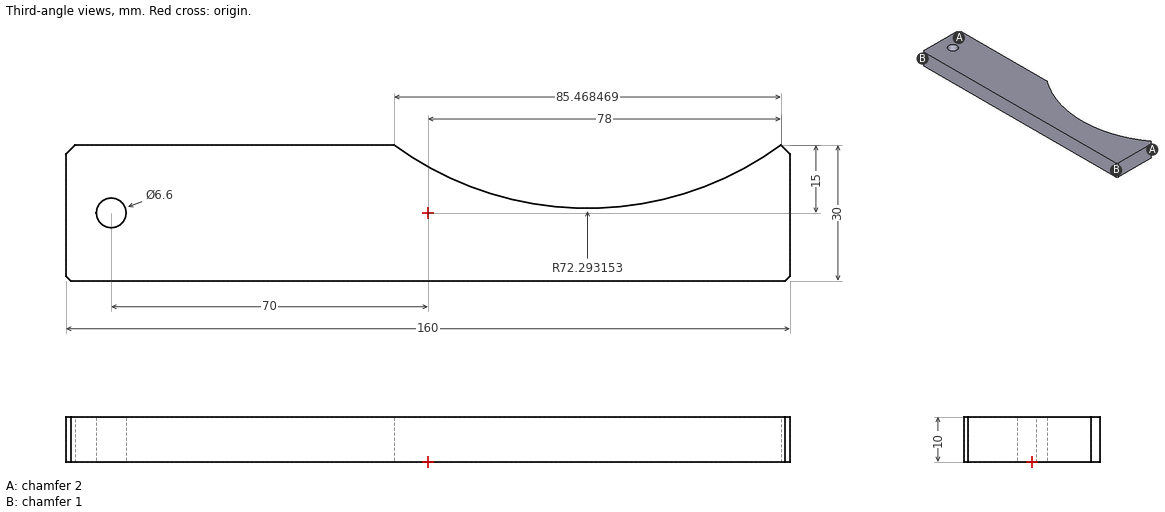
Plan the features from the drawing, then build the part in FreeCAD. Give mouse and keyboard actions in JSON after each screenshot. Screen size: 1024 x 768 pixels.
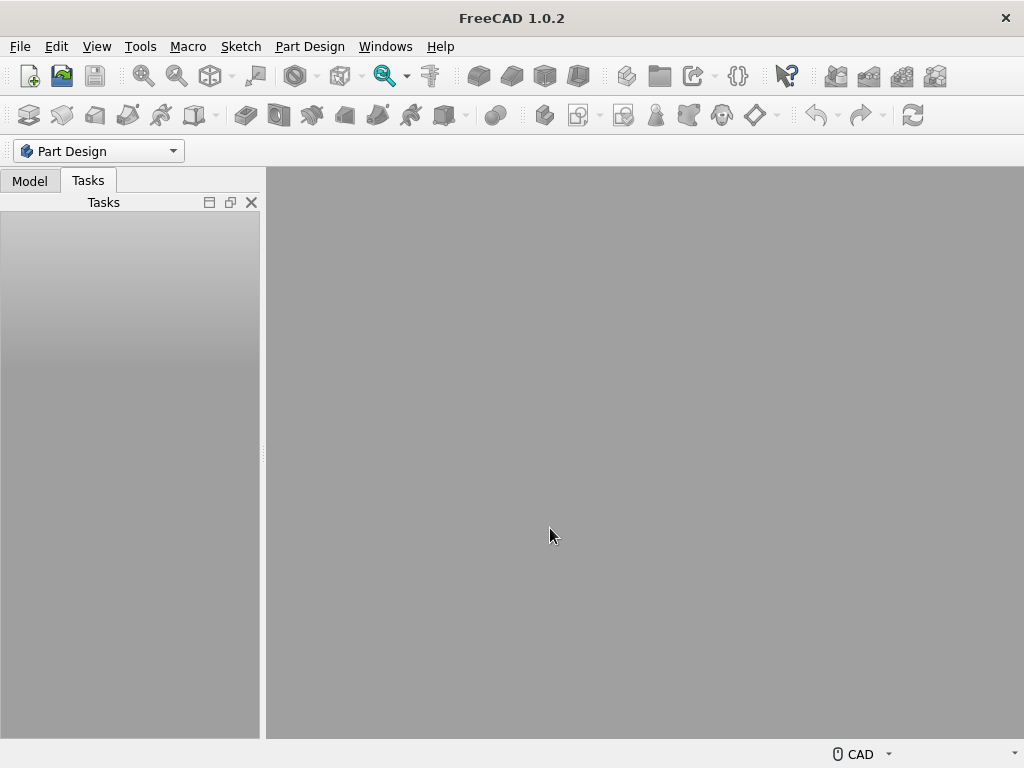
{"action": "left_click", "coordinate": [29, 76]}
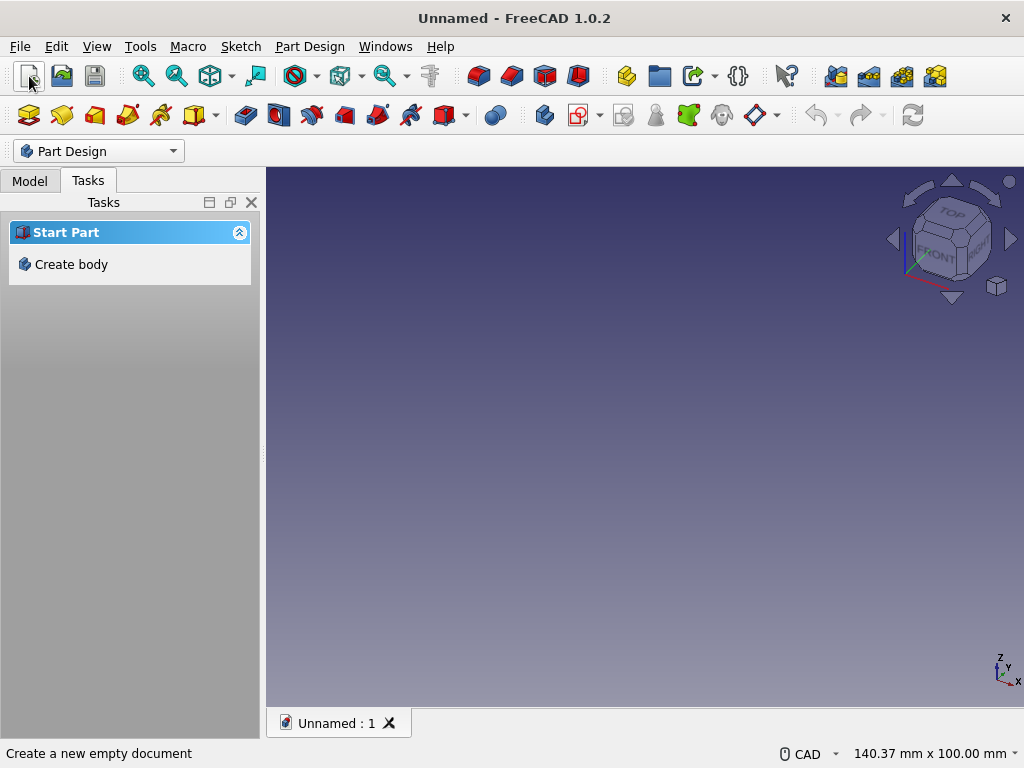
{"action": "left_click", "coordinate": [578, 116]}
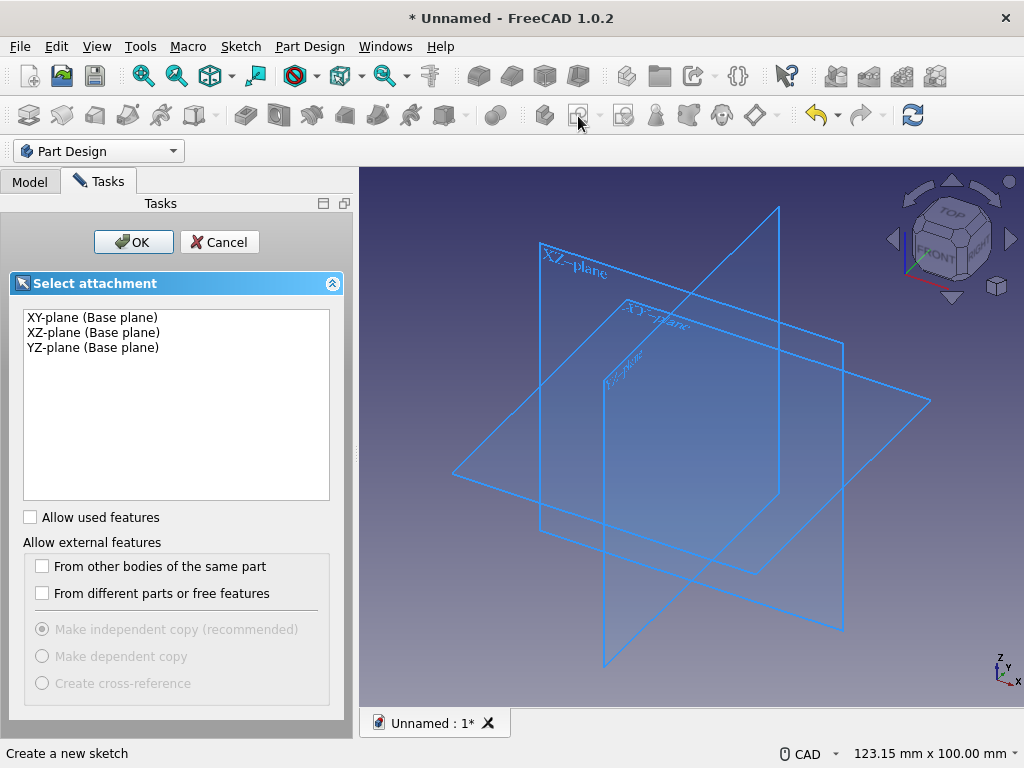
{"action": "left_click", "coordinate": [84, 318]}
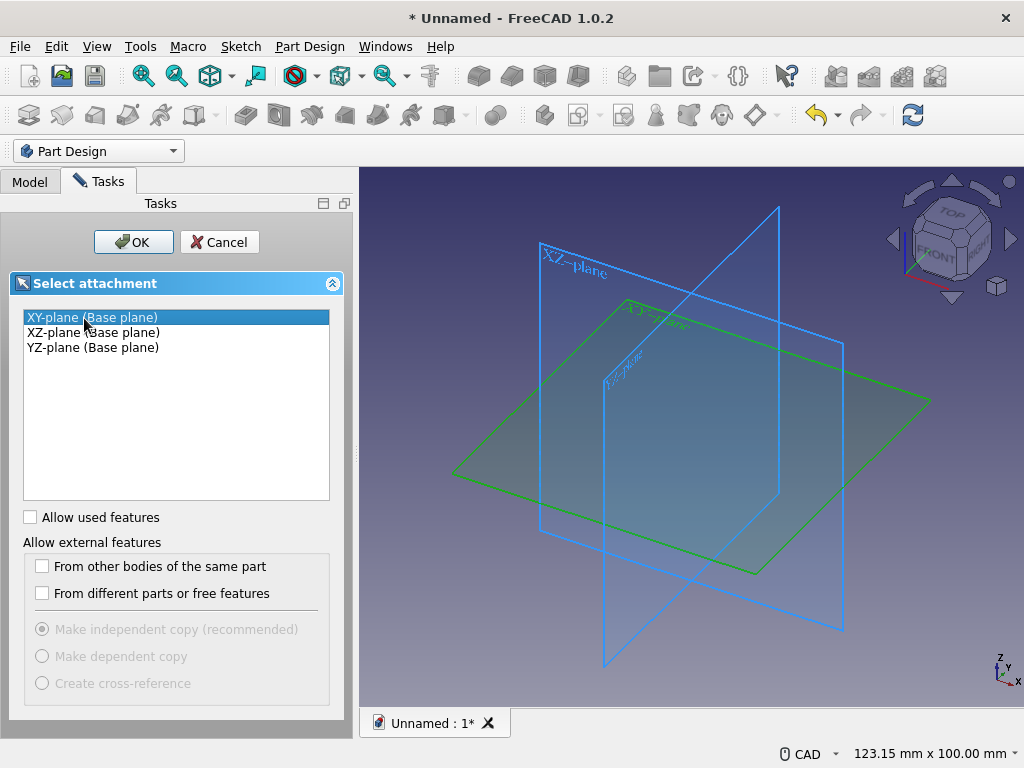
{"action": "left_click", "coordinate": [134, 242]}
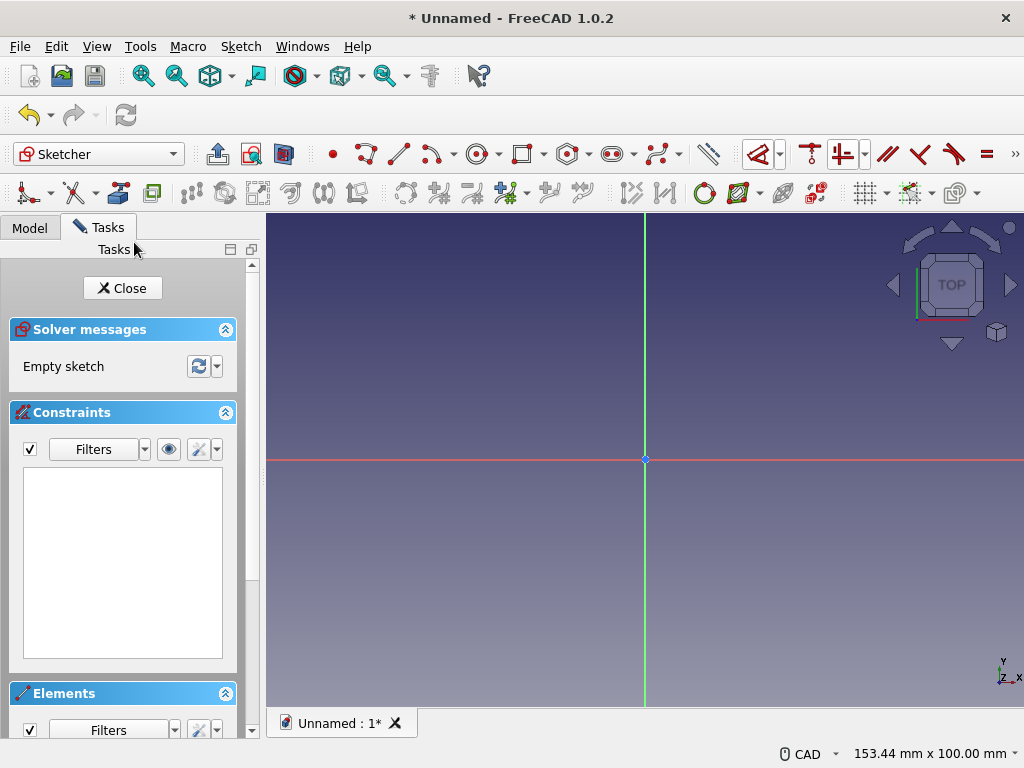
{"action": "scroll", "coordinate": [493, 460], "scroll_direction": "down", "scroll_amount": 3}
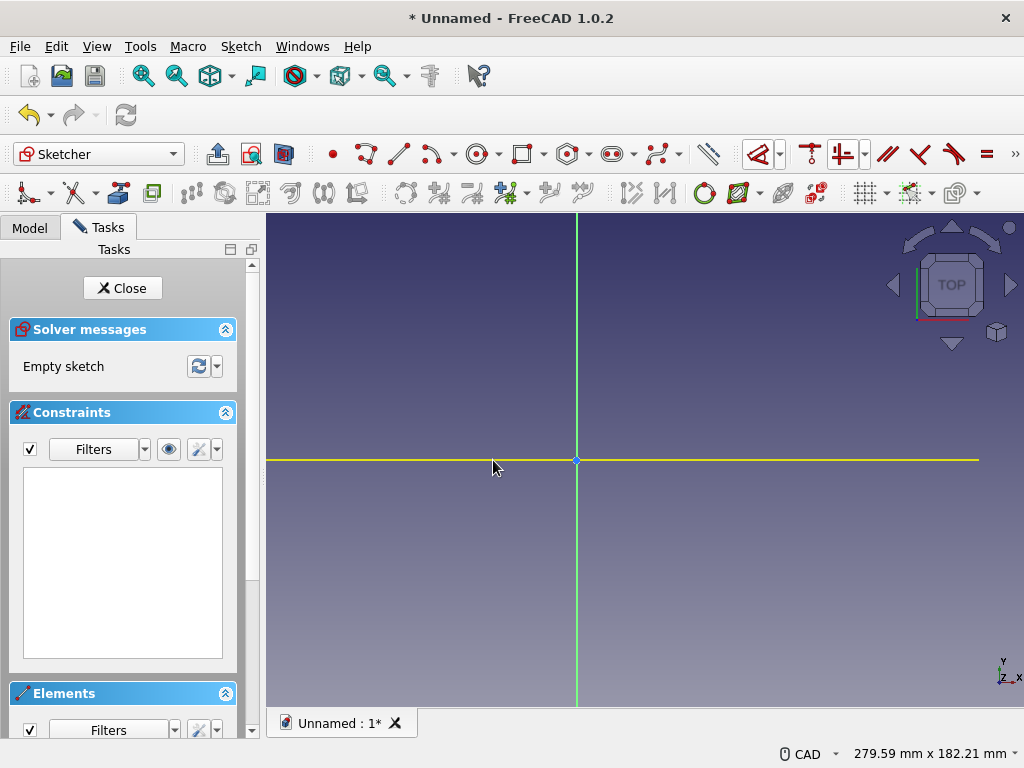
{"action": "key", "text": "g v"}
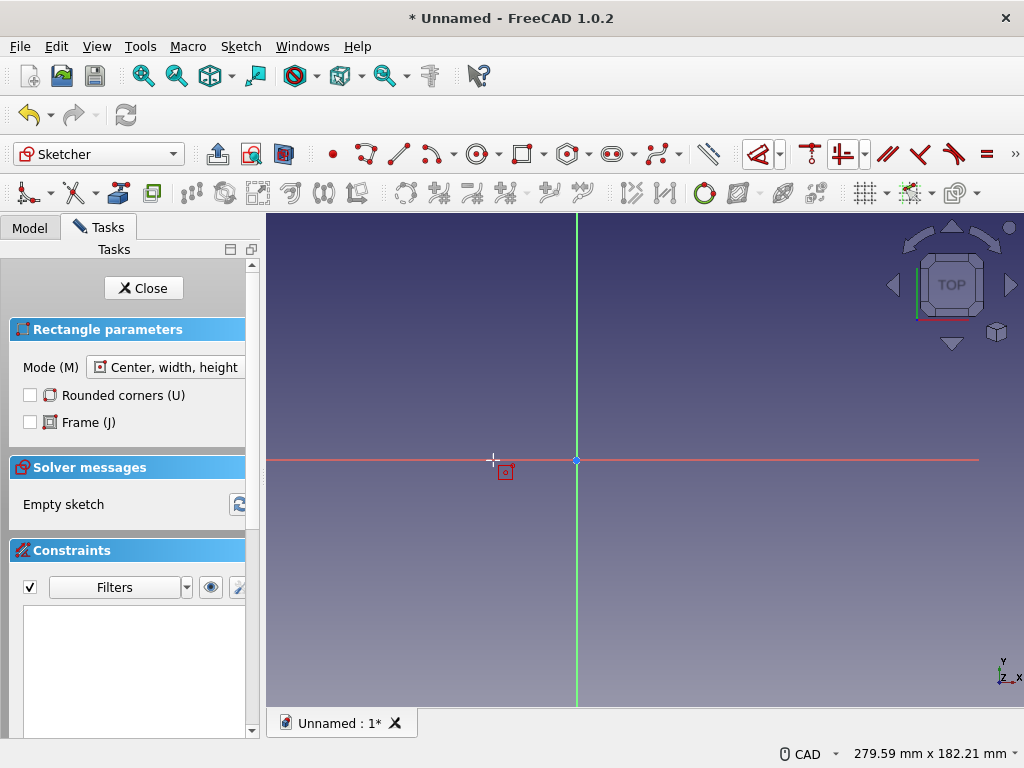
{"action": "left_click", "coordinate": [577, 460]}
{"action": "mouse_move", "coordinate": [793, 420]}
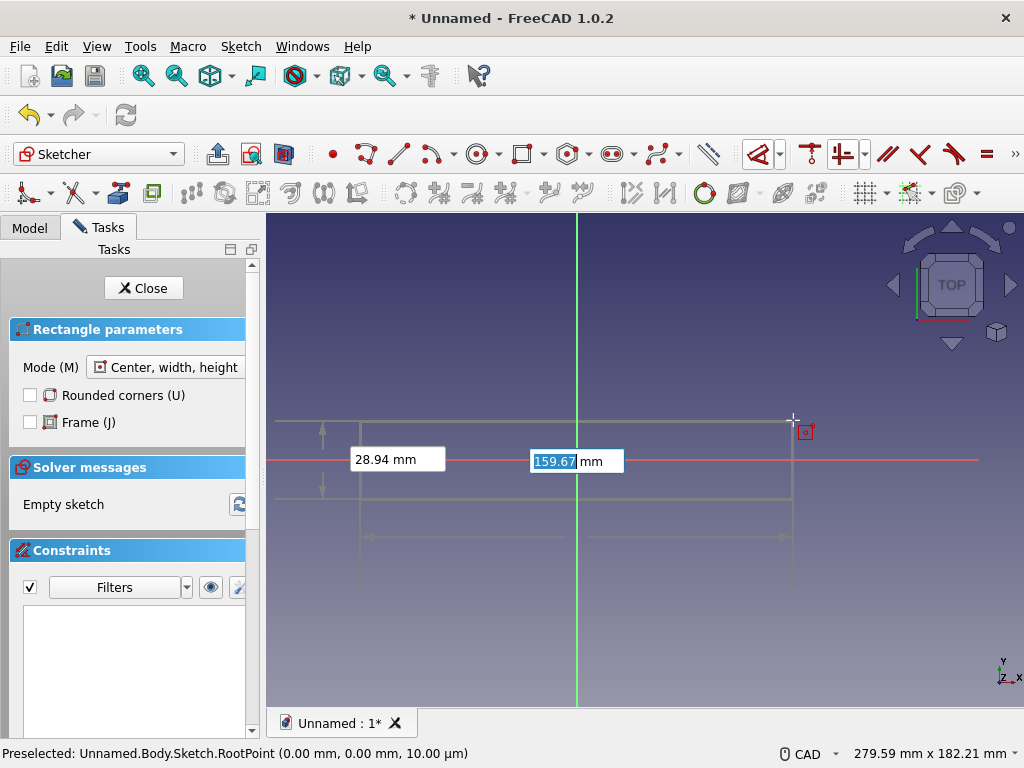
{"action": "type", "text": "160"}
{"action": "key", "text": "Tab"}
{"action": "type", "text": "30"}
{"action": "key", "text": "Return"}
{"action": "key", "text": "Escape"}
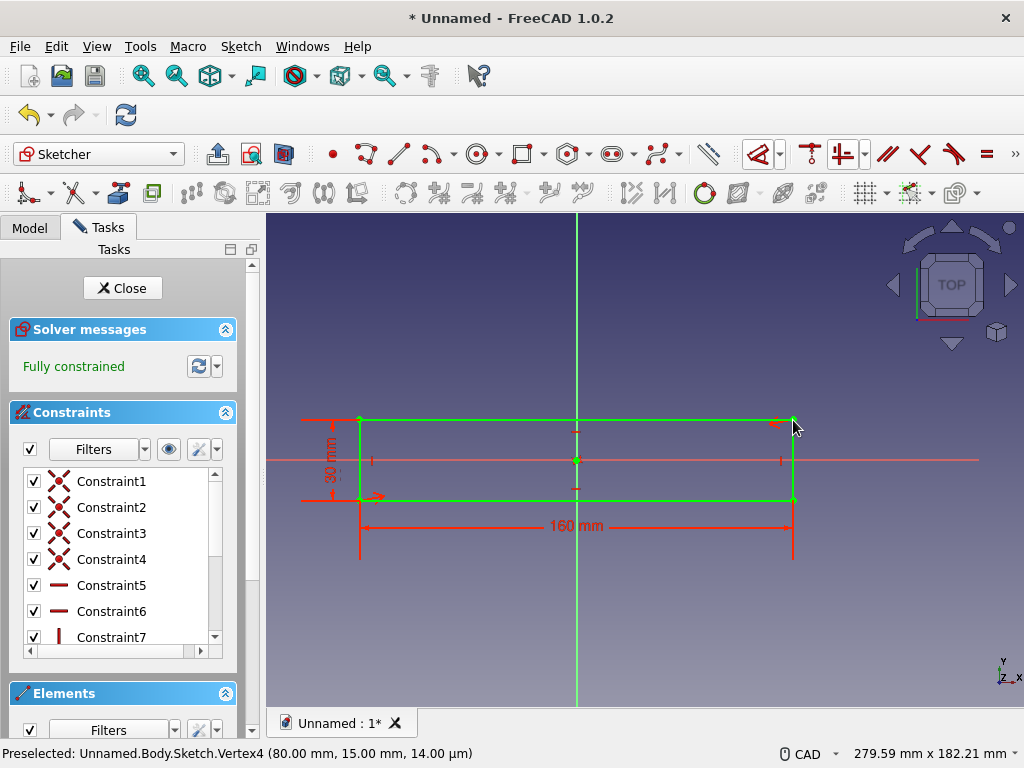
{"action": "left_click", "coordinate": [123, 288]}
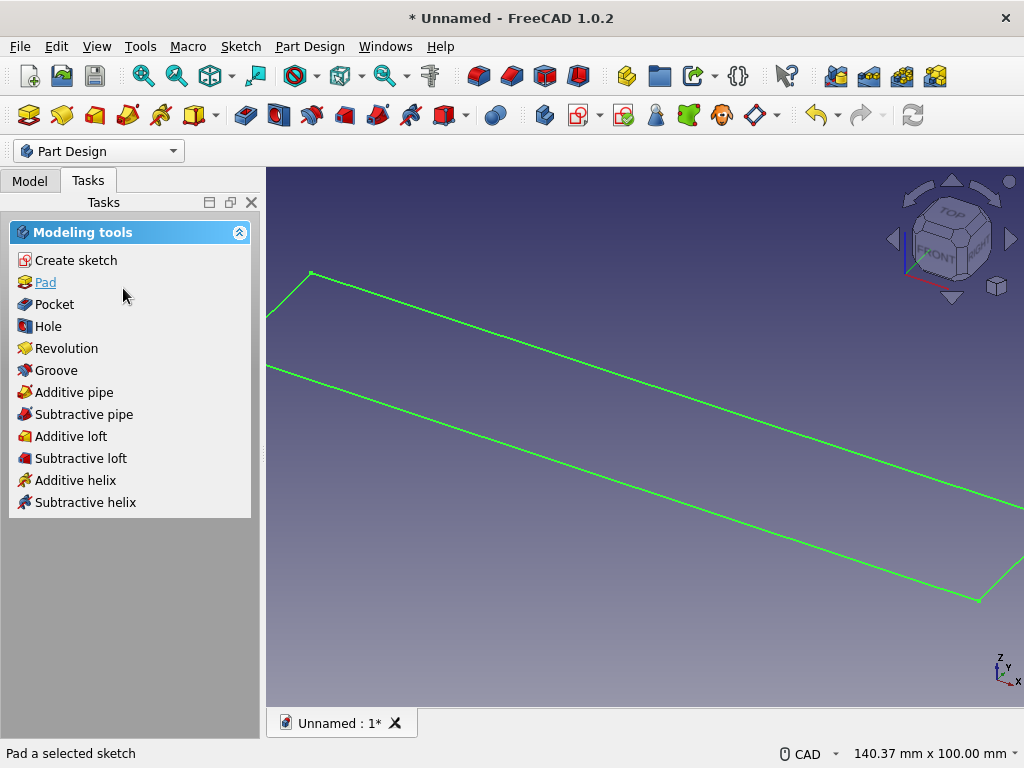
{"action": "left_click", "coordinate": [29, 116]}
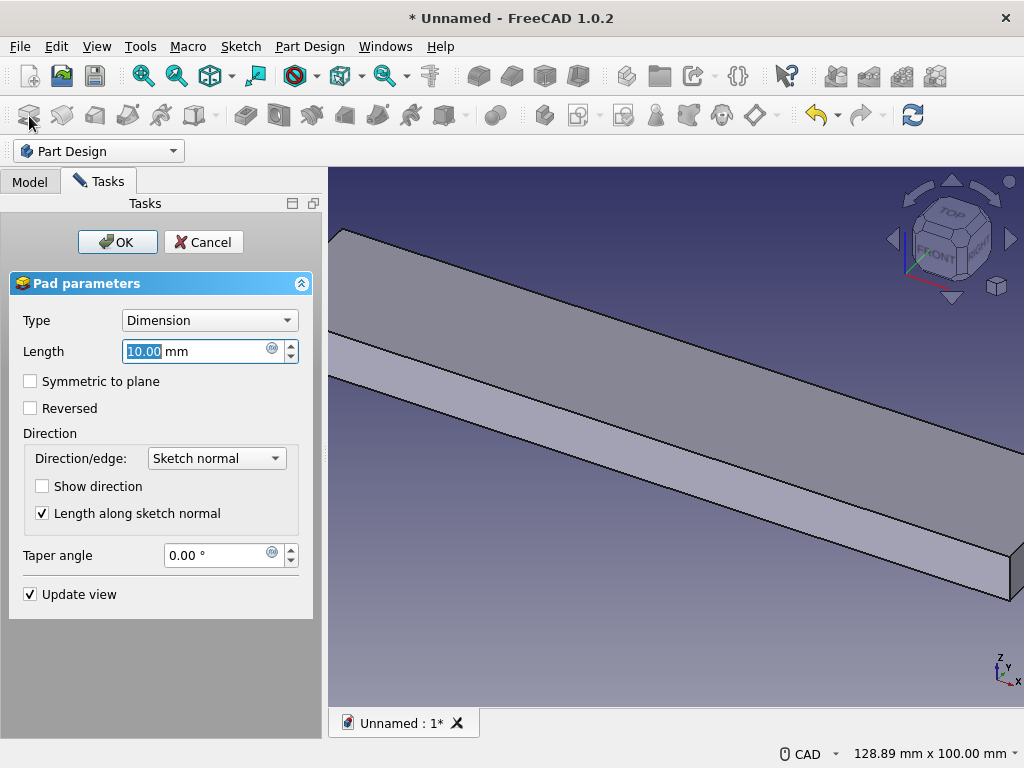
{"action": "type", "text": "10"}
{"action": "key", "text": "Tab"}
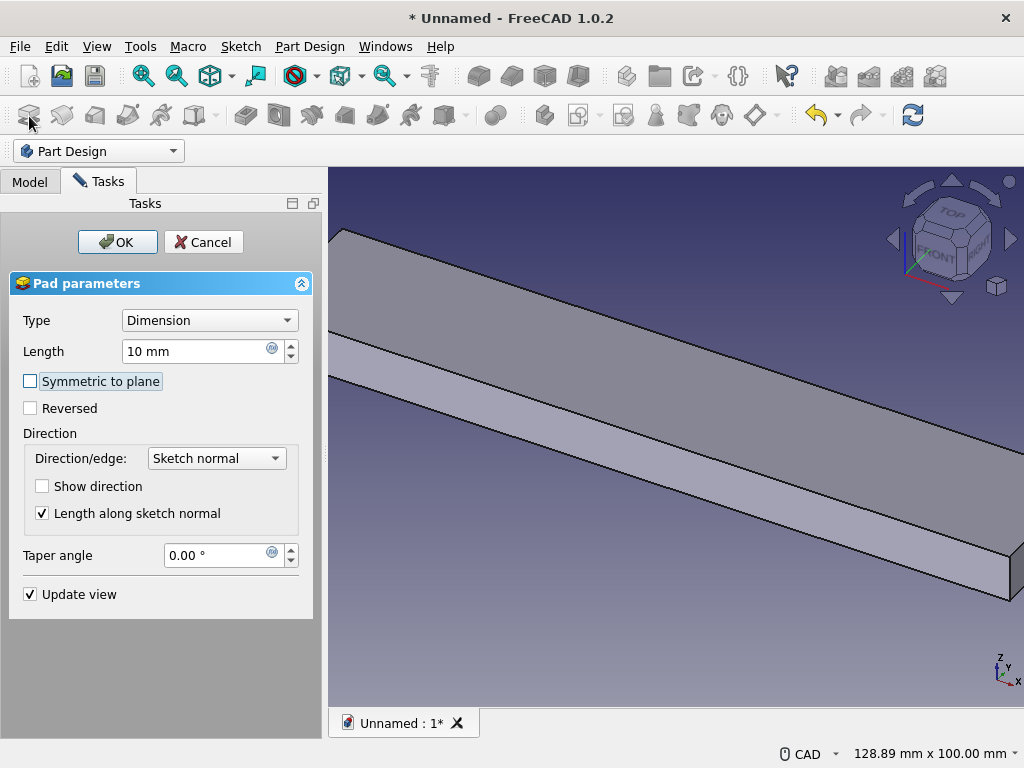
{"action": "left_click", "coordinate": [118, 242]}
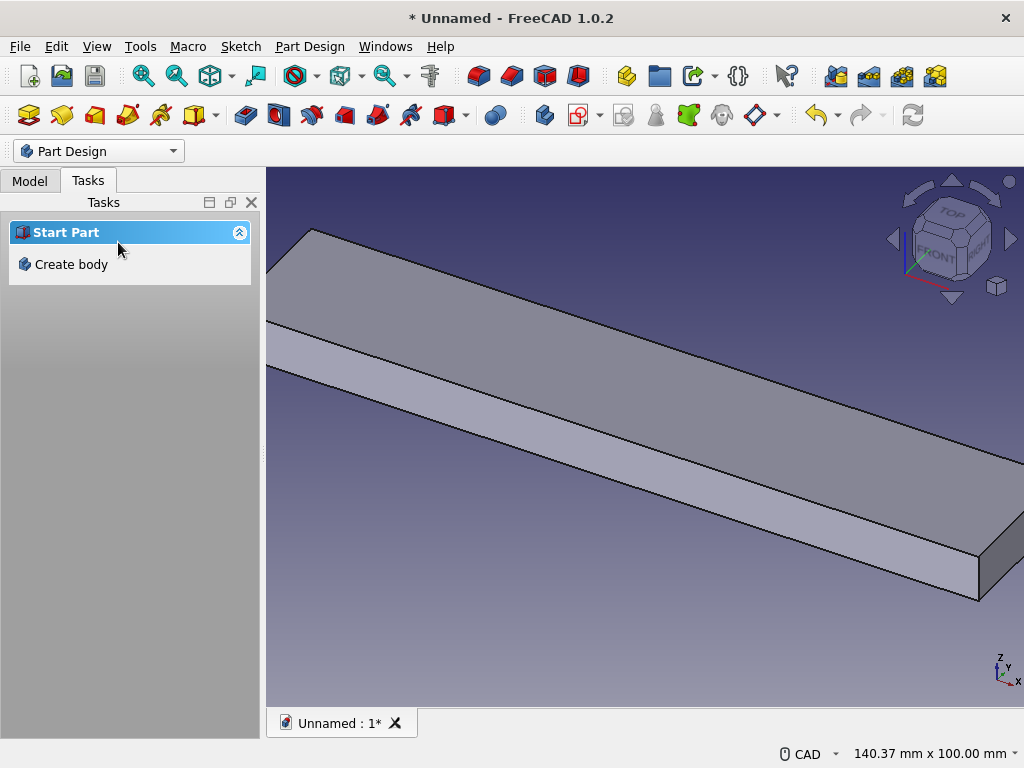
{"action": "left_click", "coordinate": [144, 76]}